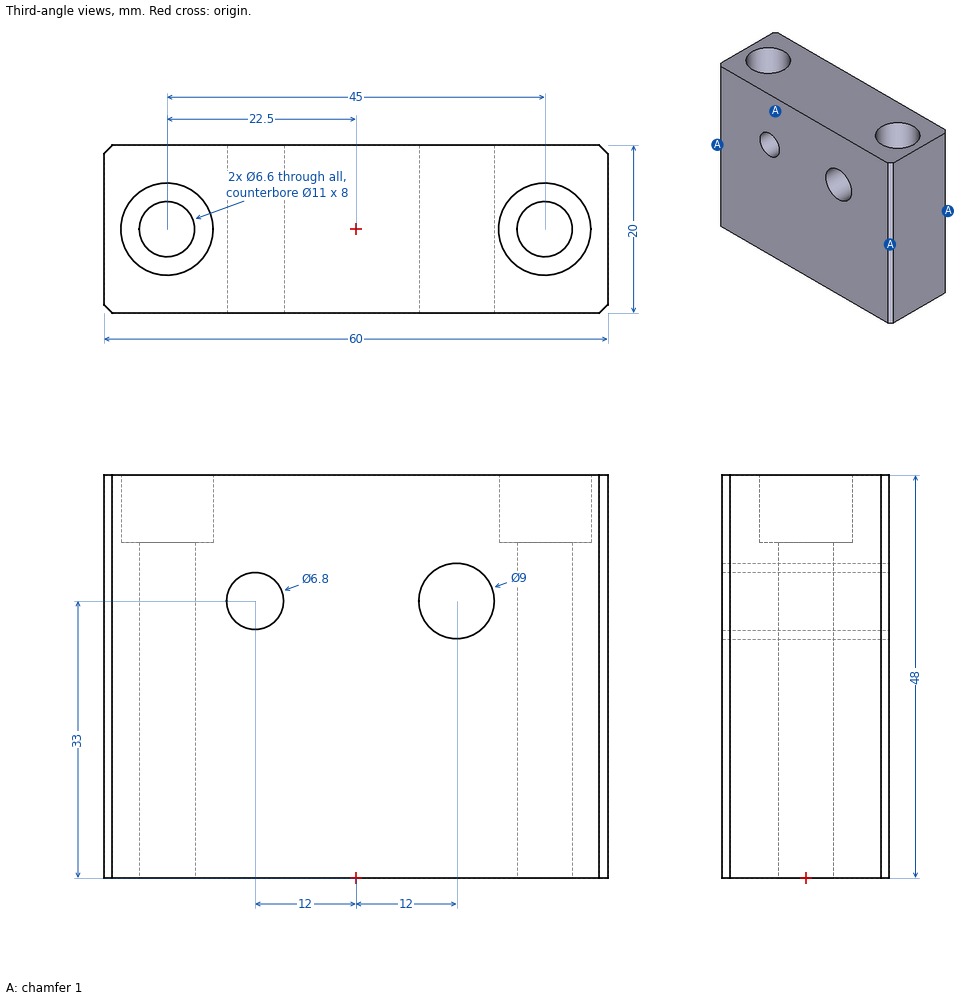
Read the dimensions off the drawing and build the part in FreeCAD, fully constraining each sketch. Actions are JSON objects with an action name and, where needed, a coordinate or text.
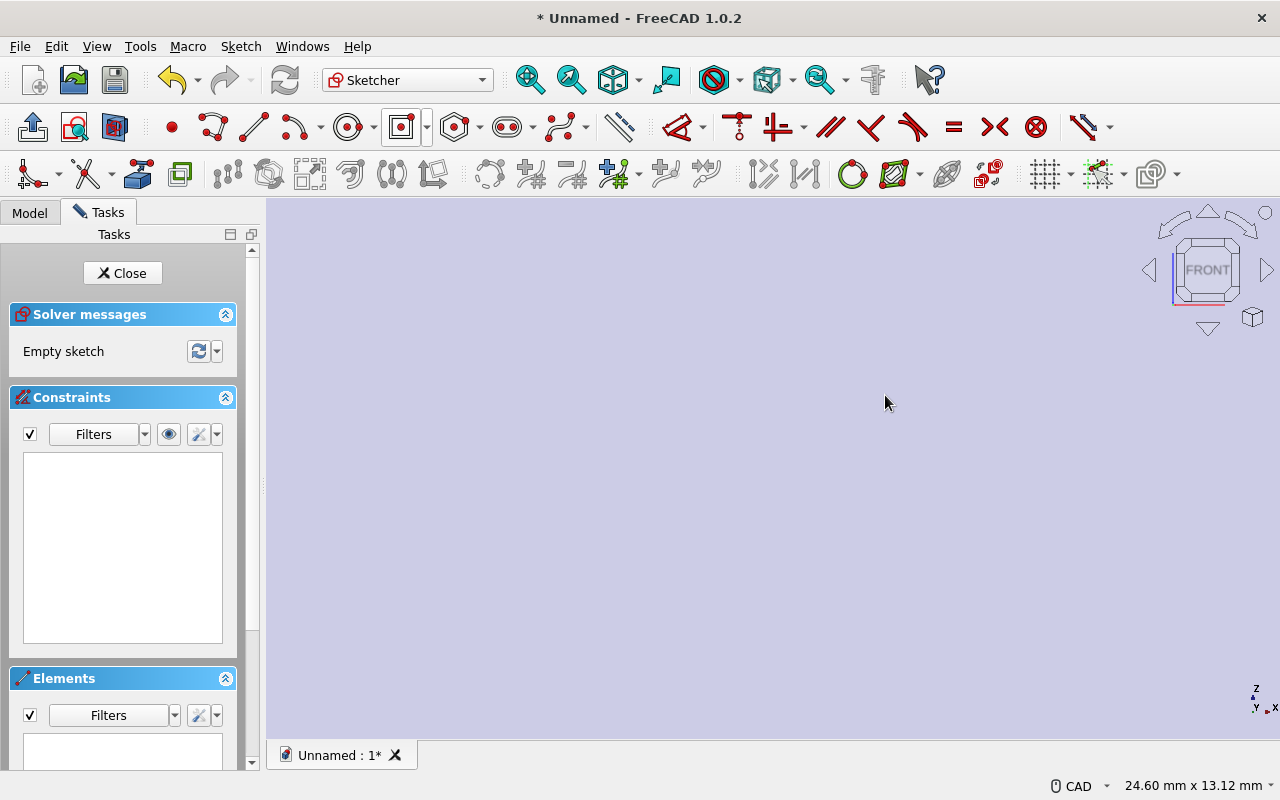
{"action": "left_click", "coordinate": [348, 128]}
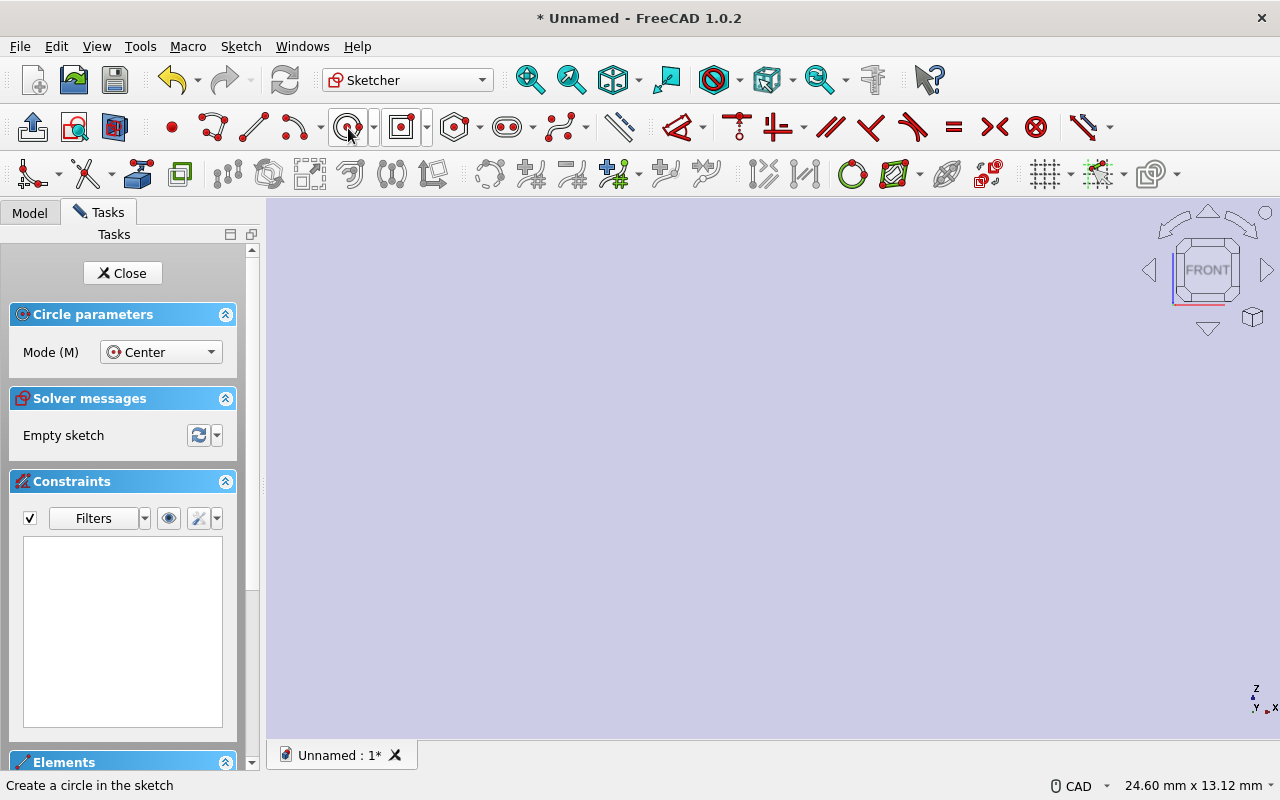
{"action": "left_click", "coordinate": [699, 467]}
{"action": "mouse_move", "coordinate": [830, 336]}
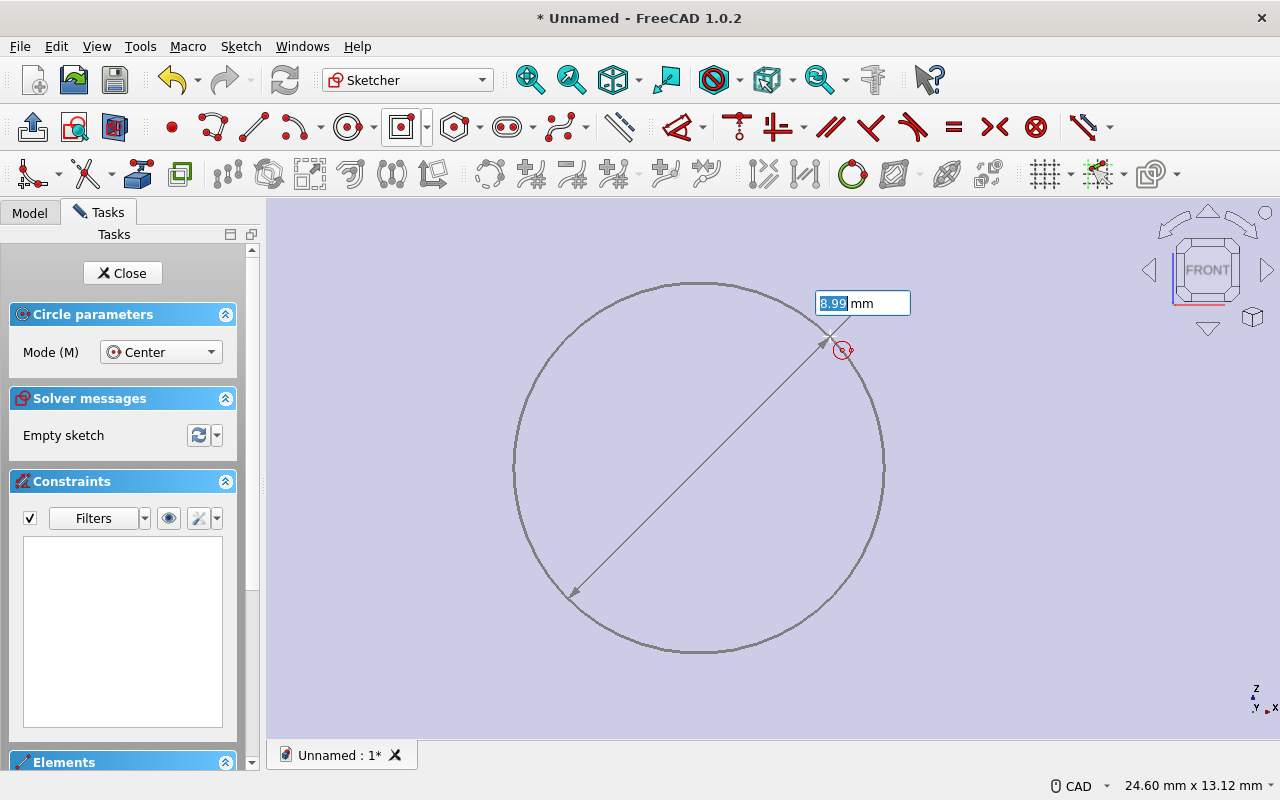
{"action": "type", "text": "9"}
{"action": "key", "text": "Return"}
{"action": "key", "text": "Escape"}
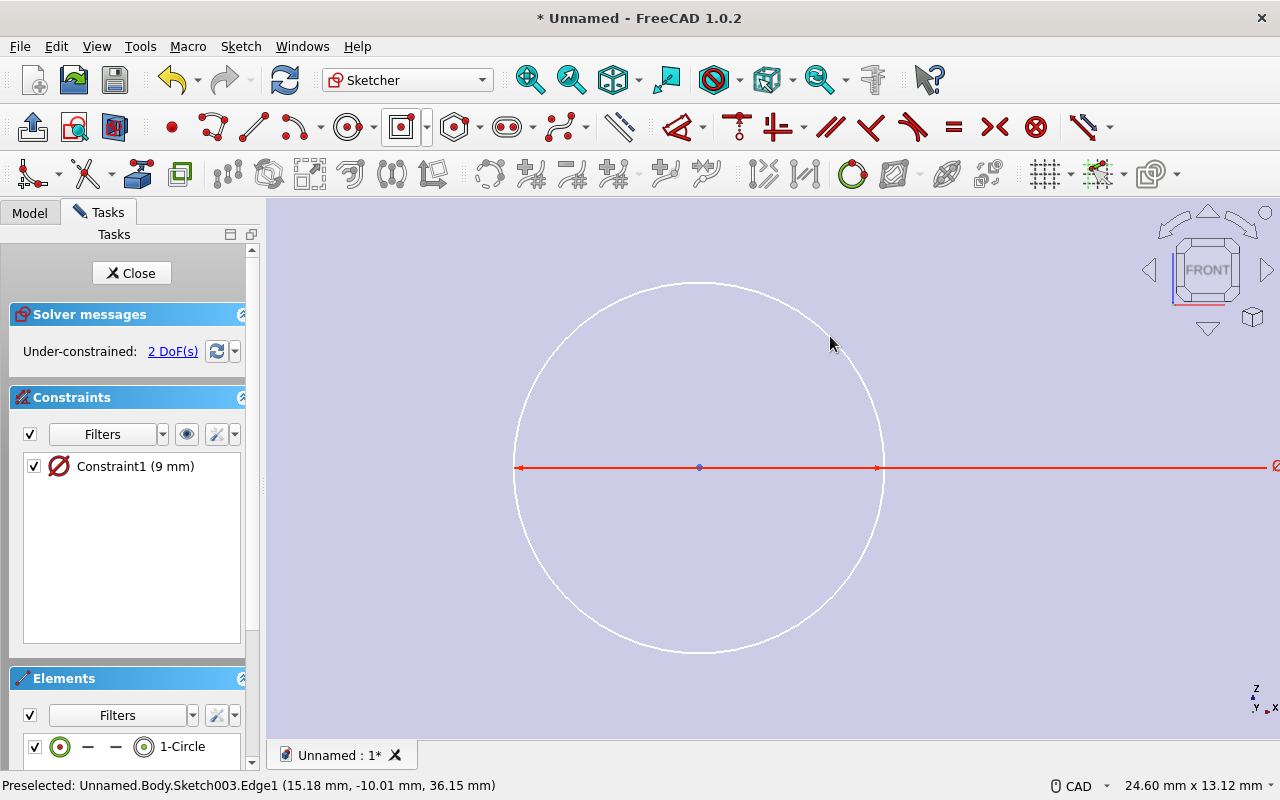
{"action": "left_click", "coordinate": [676, 128]}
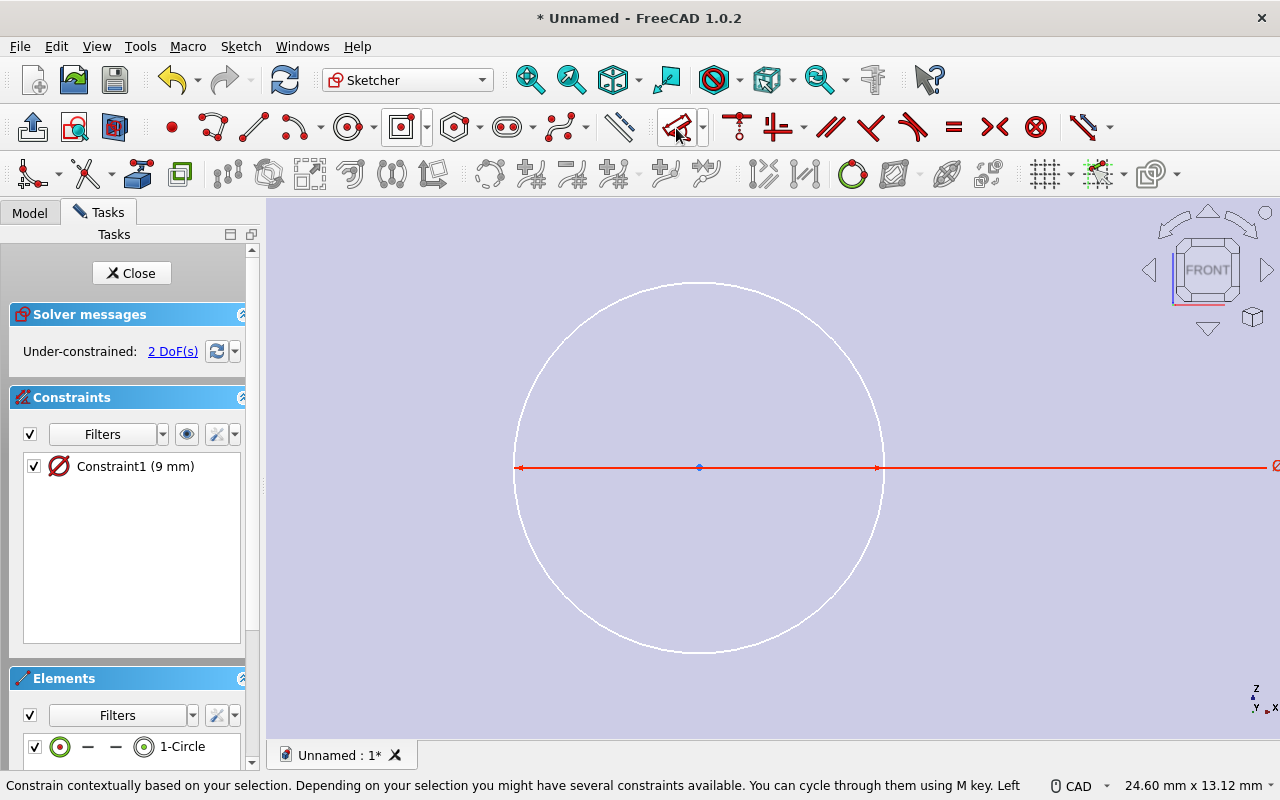
{"action": "left_click", "coordinate": [699, 468]}
{"action": "left_click", "coordinate": [496, 434]}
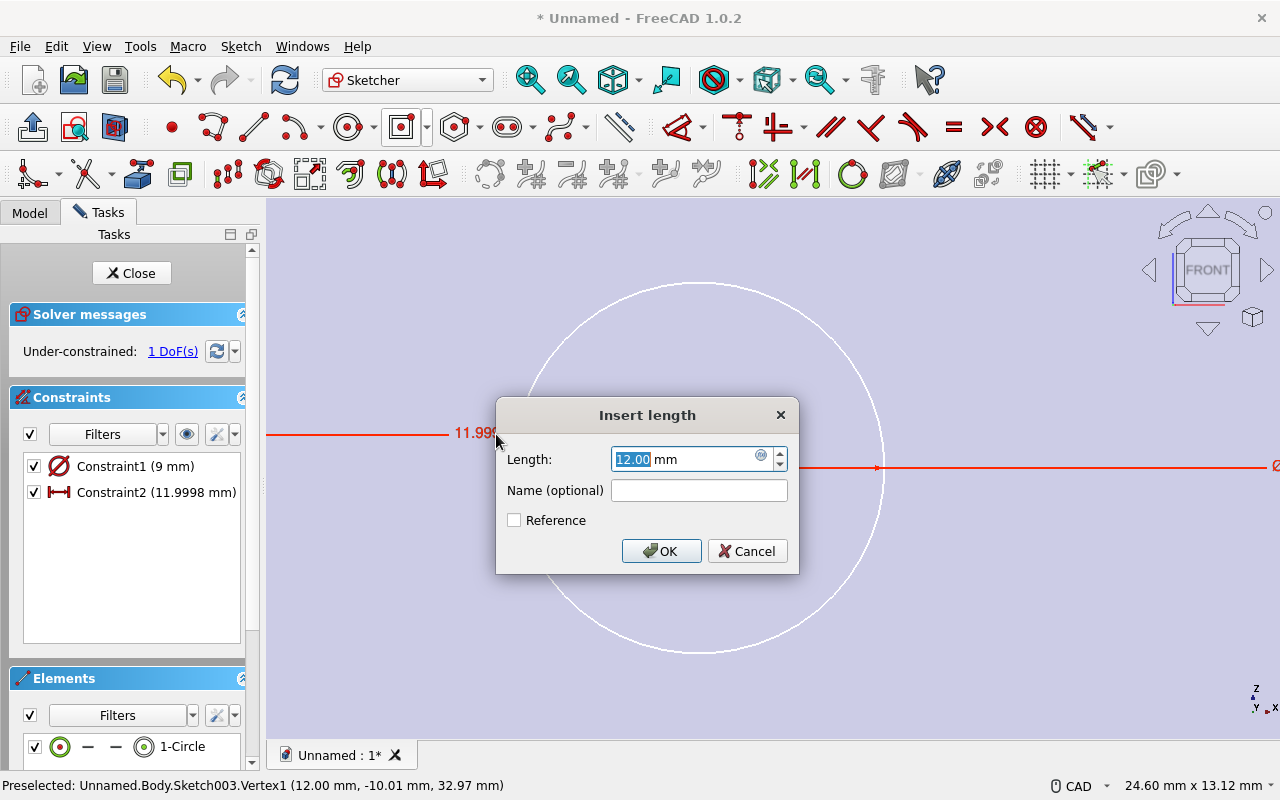
{"action": "type", "text": "12"}
{"action": "key", "text": "Return"}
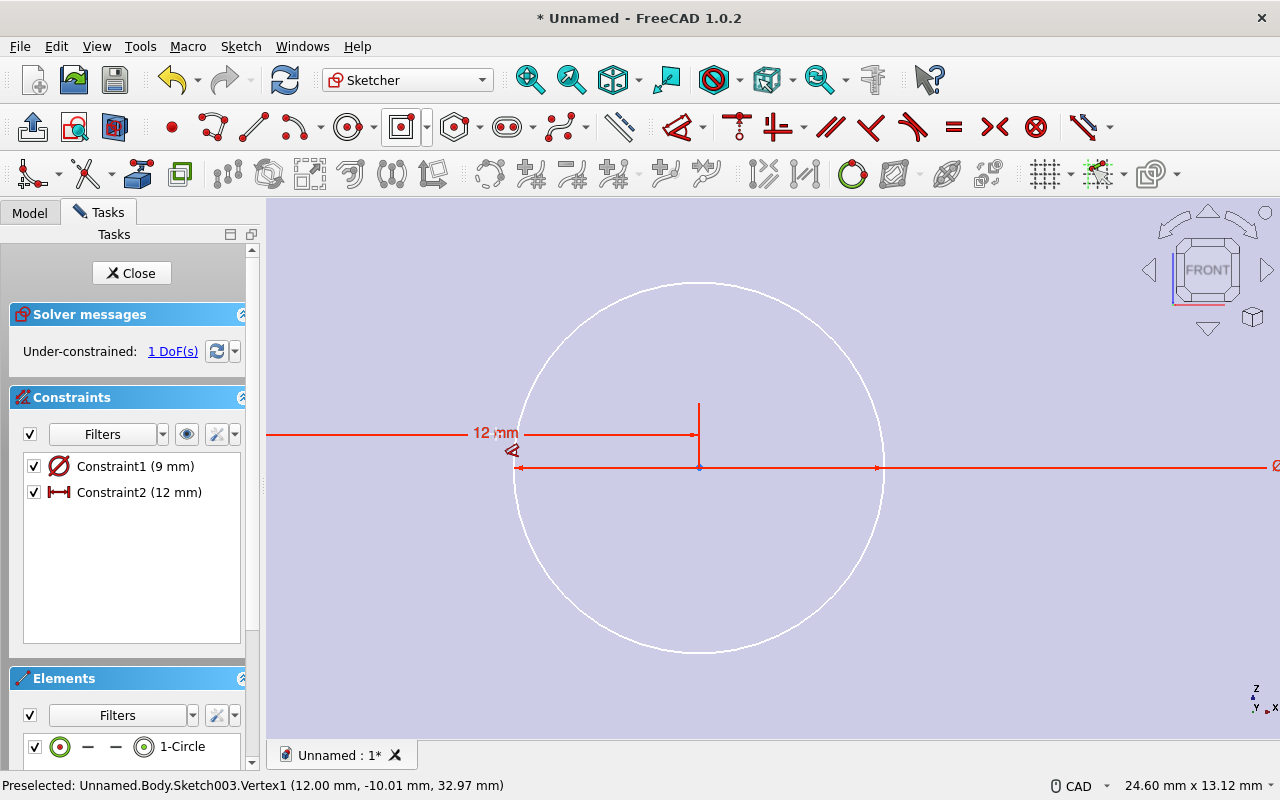
{"action": "left_click", "coordinate": [699, 468]}
{"action": "left_click", "coordinate": [733, 589]}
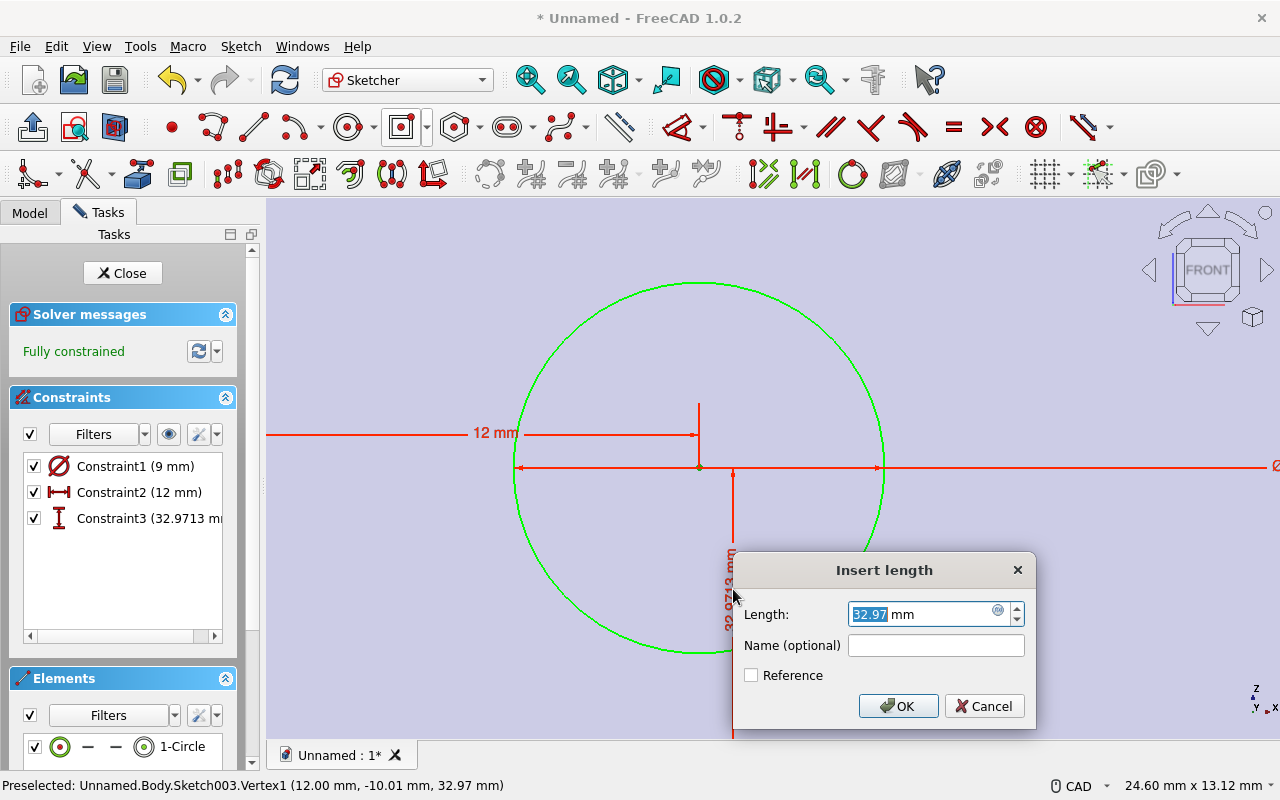
{"action": "type", "text": "33"}
{"action": "key", "text": "Return"}
{"action": "key", "text": "Escape"}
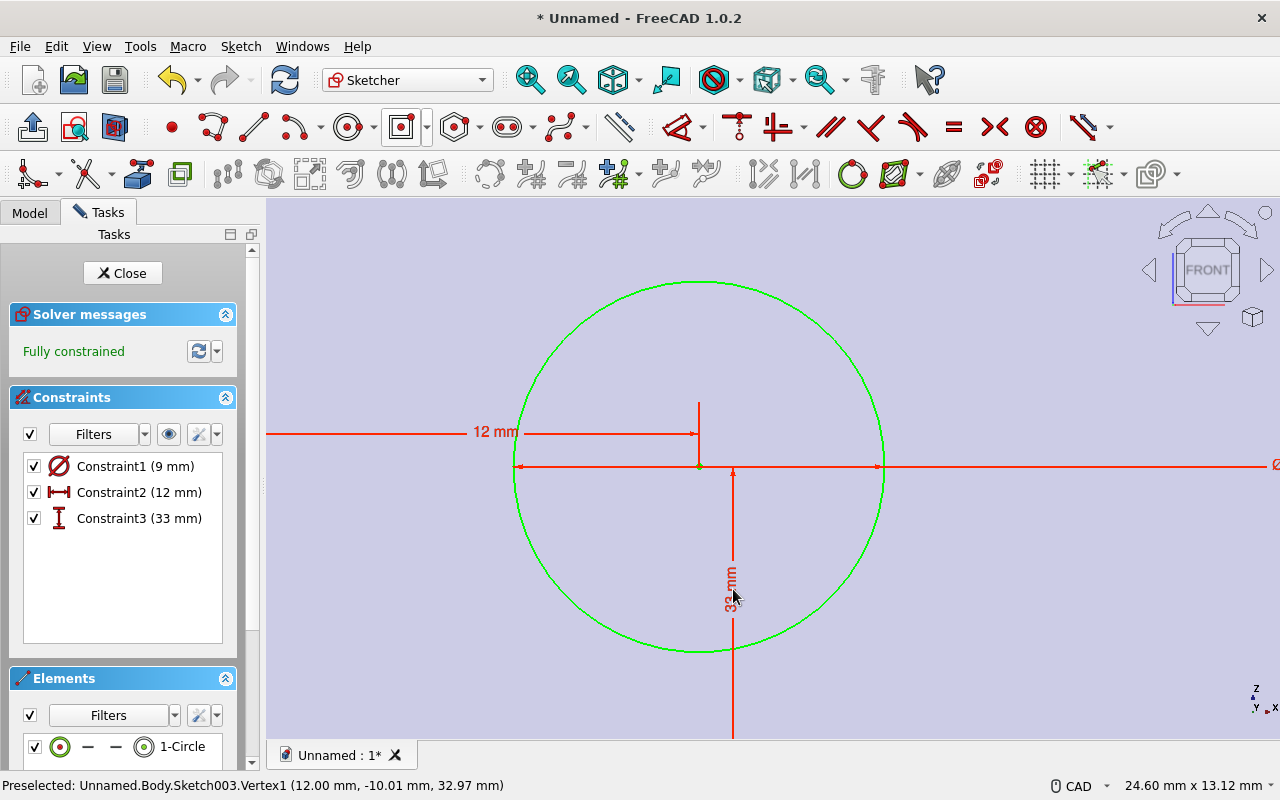
{"action": "left_click", "coordinate": [123, 273]}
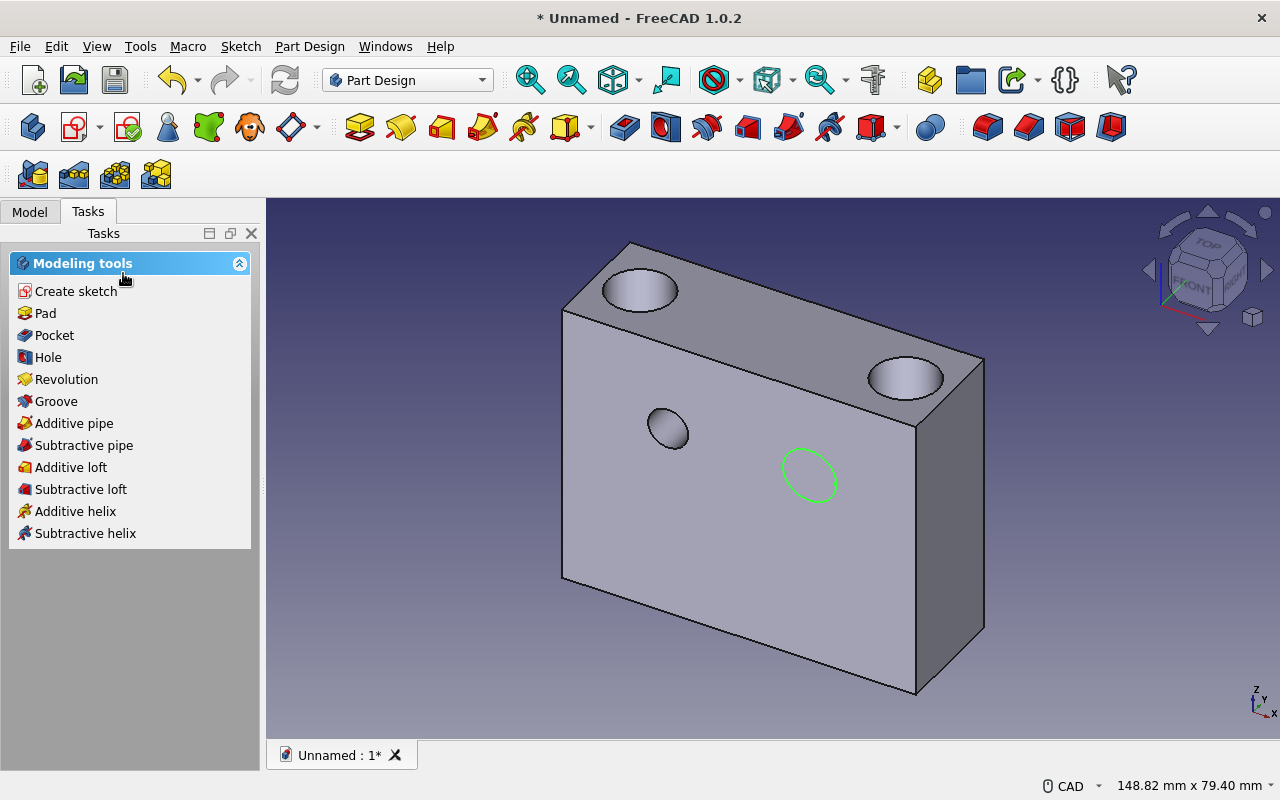
{"action": "left_click", "coordinate": [625, 128]}